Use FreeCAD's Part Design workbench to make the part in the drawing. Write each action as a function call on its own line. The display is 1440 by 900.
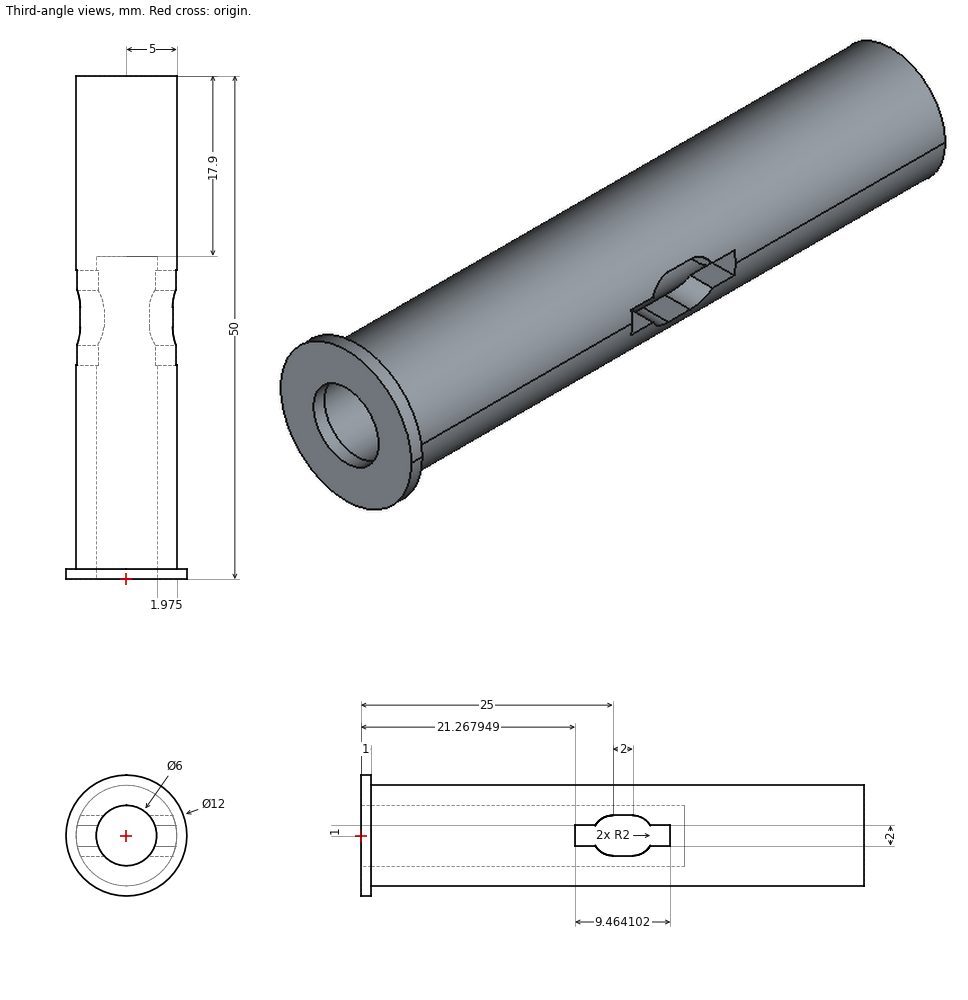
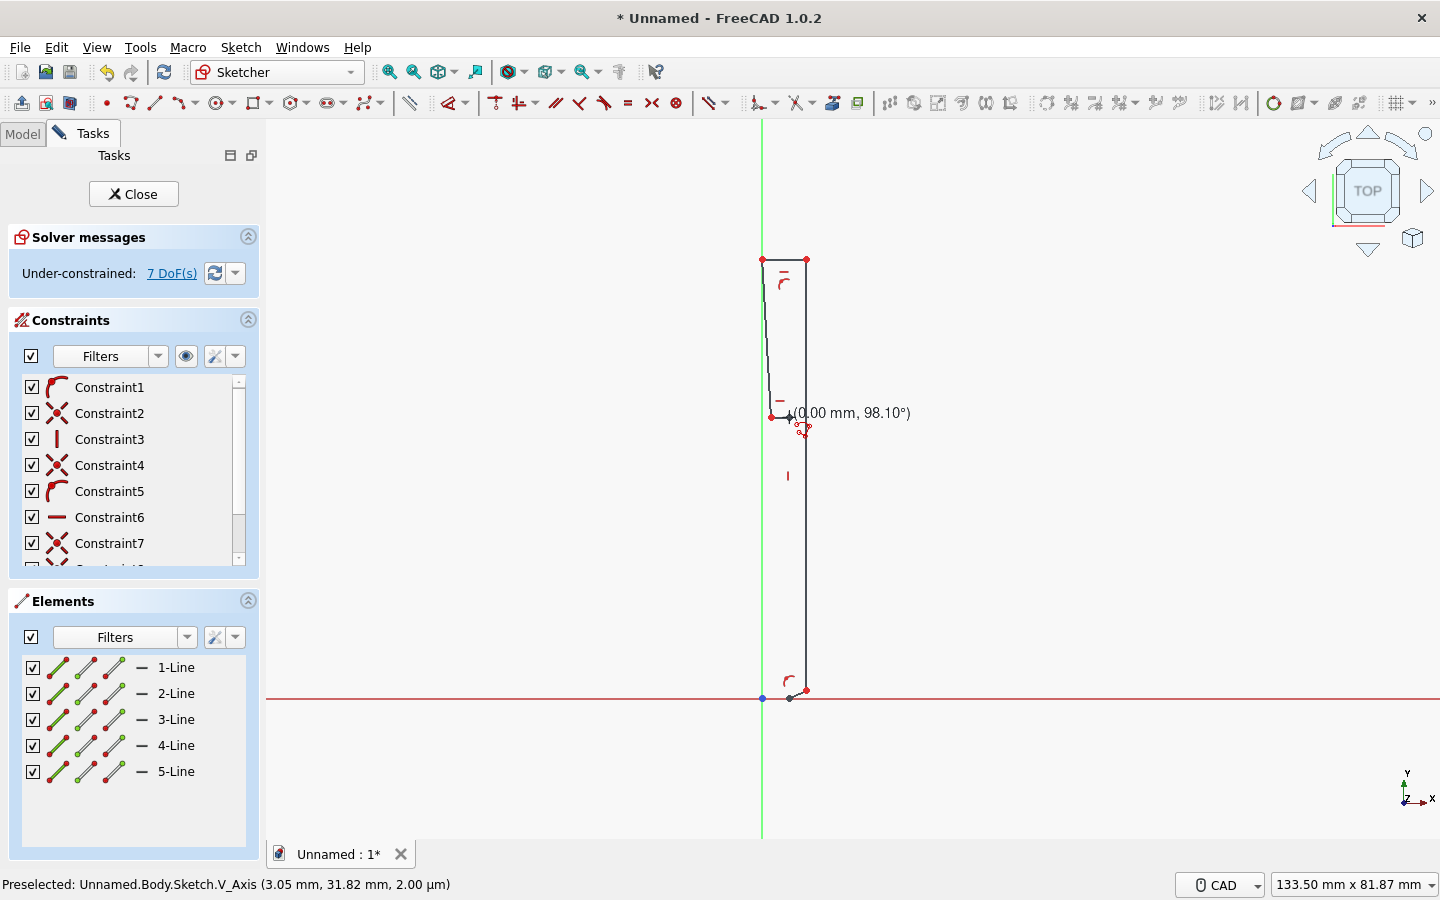
scroll(789, 699, up, 4)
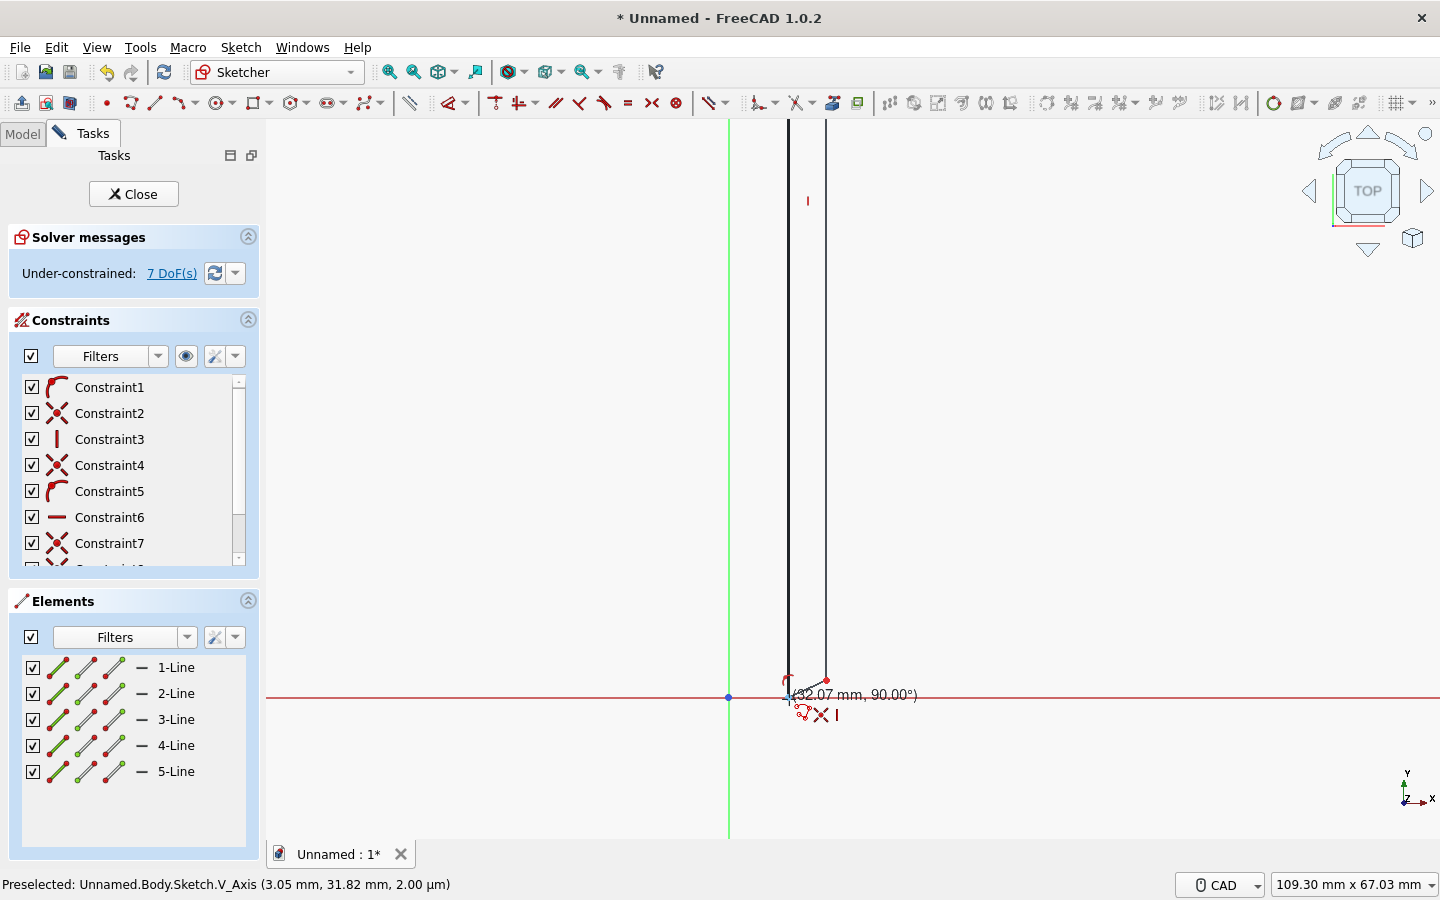
click(788, 698)
key(Escape)
key(Escape)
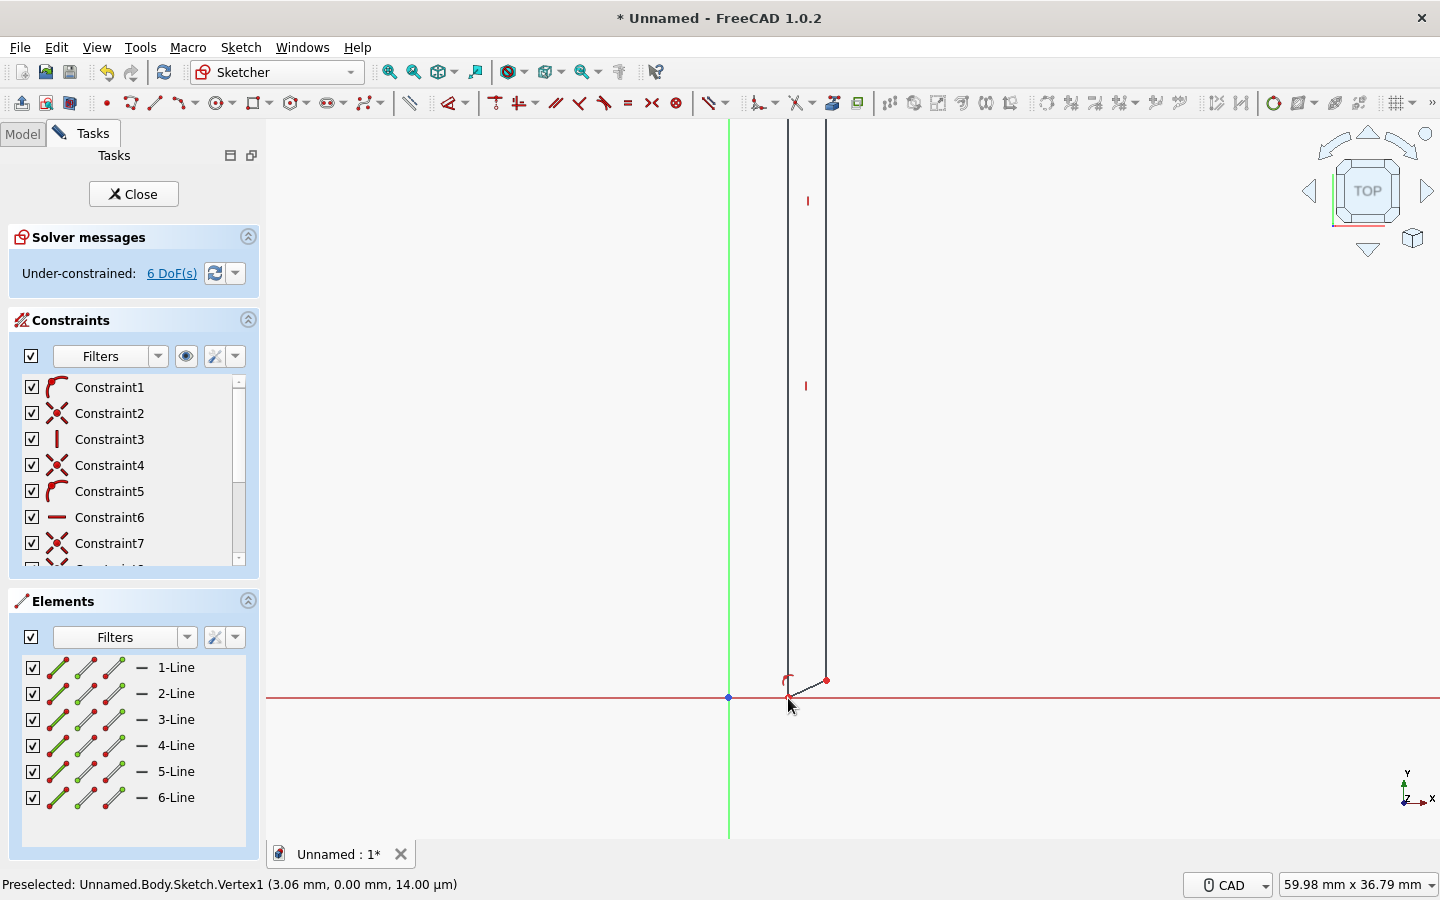
click(815, 685)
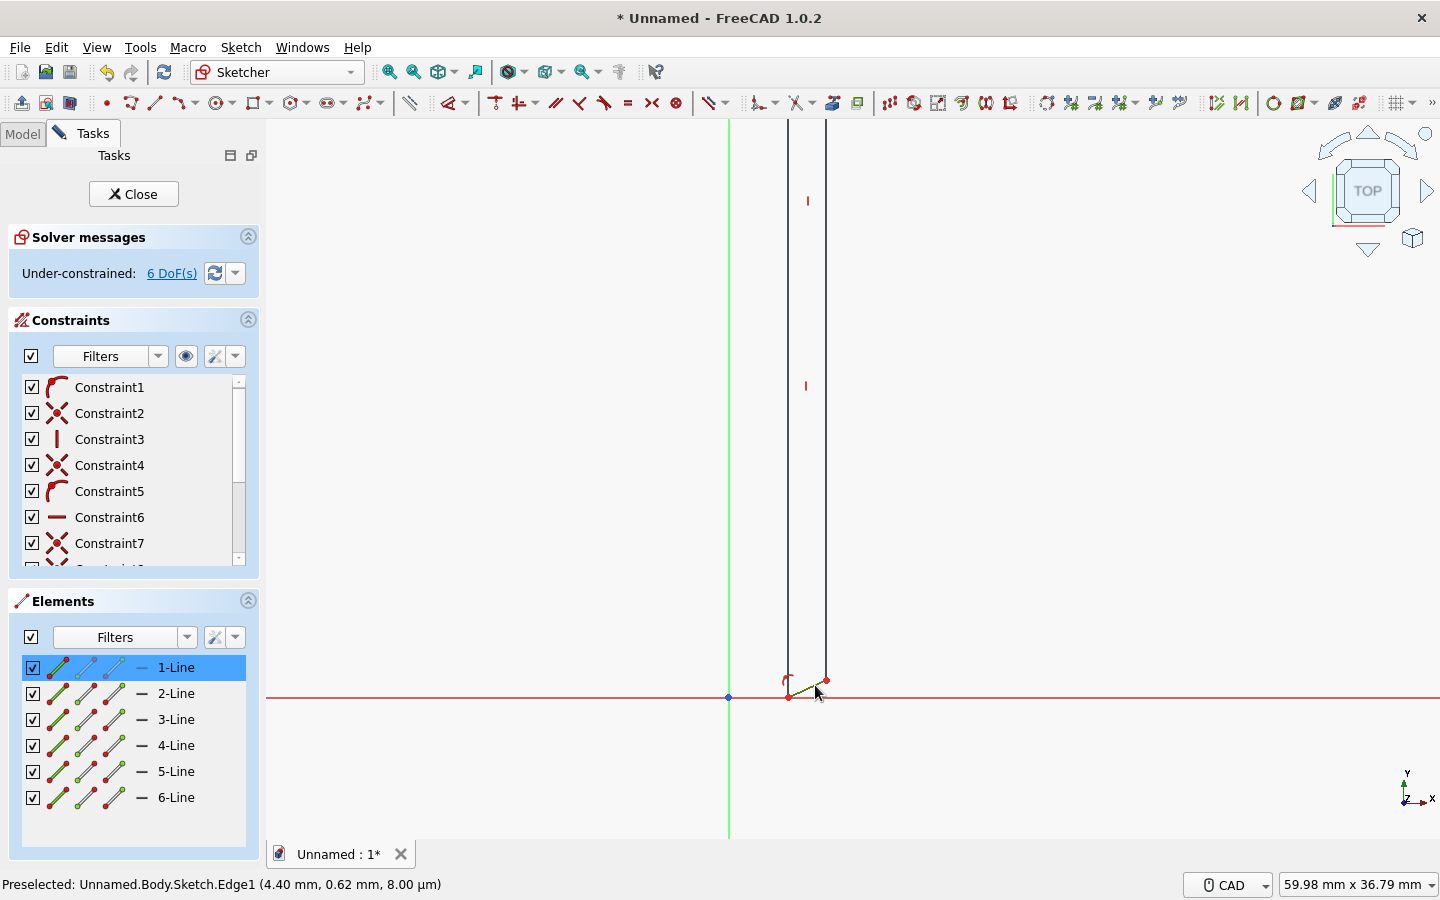
key(h)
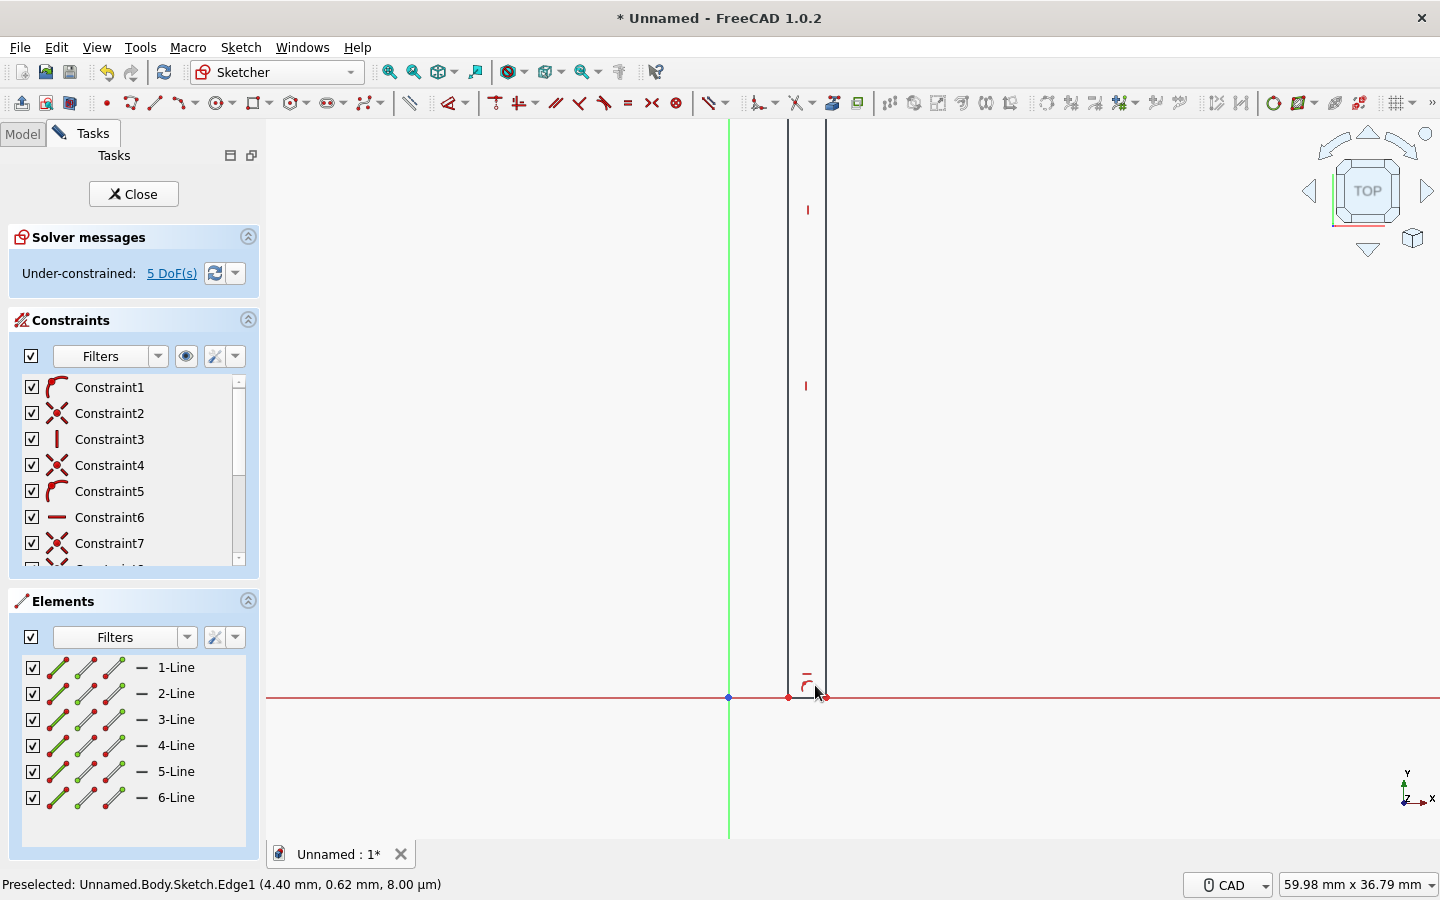
scroll(790, 700, down, 4)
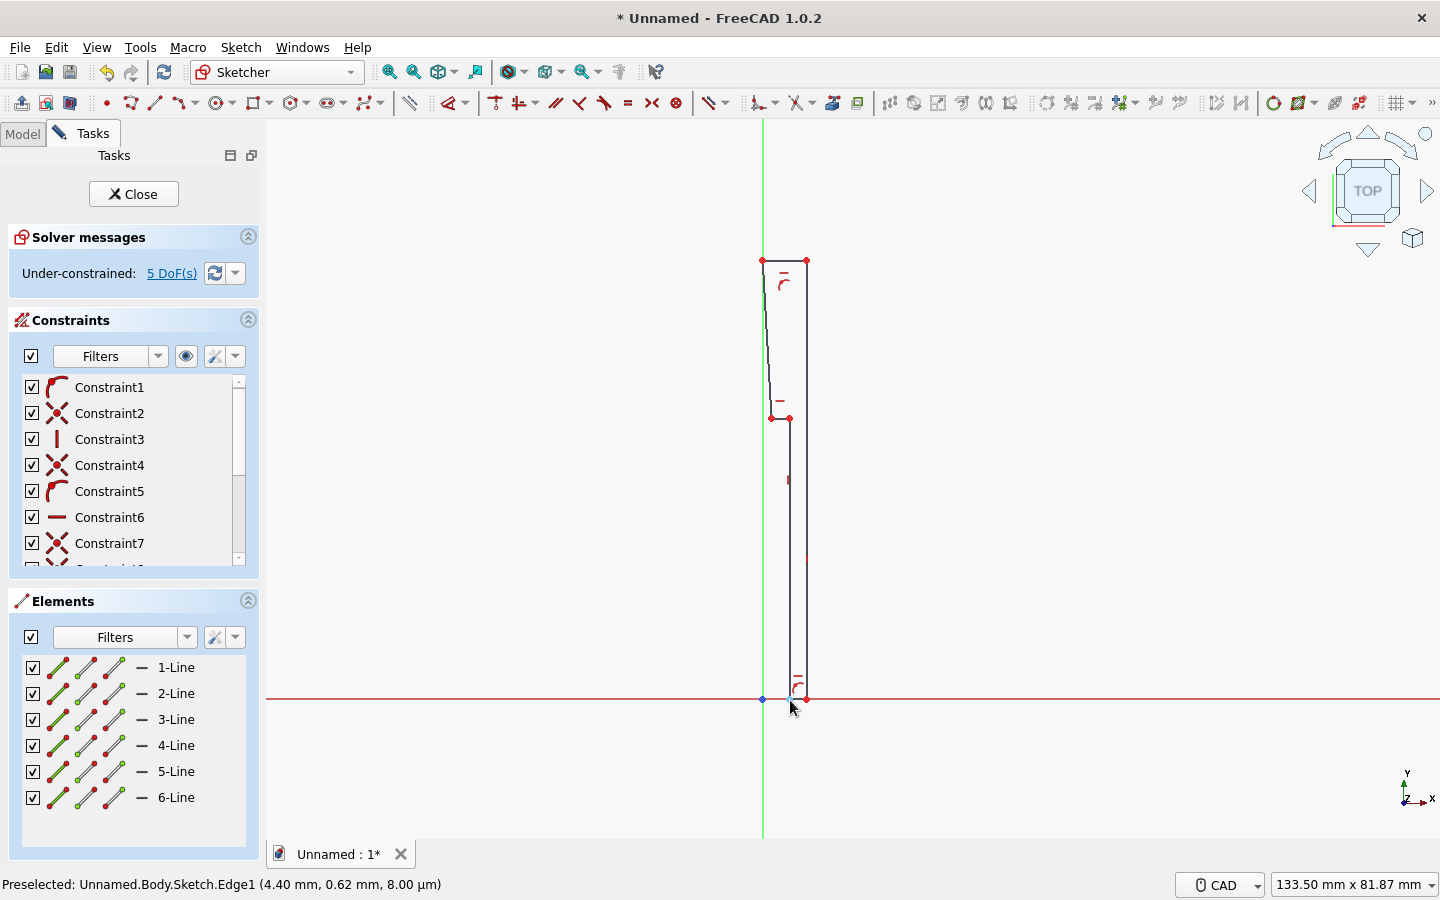
scroll(769, 371, up, 4)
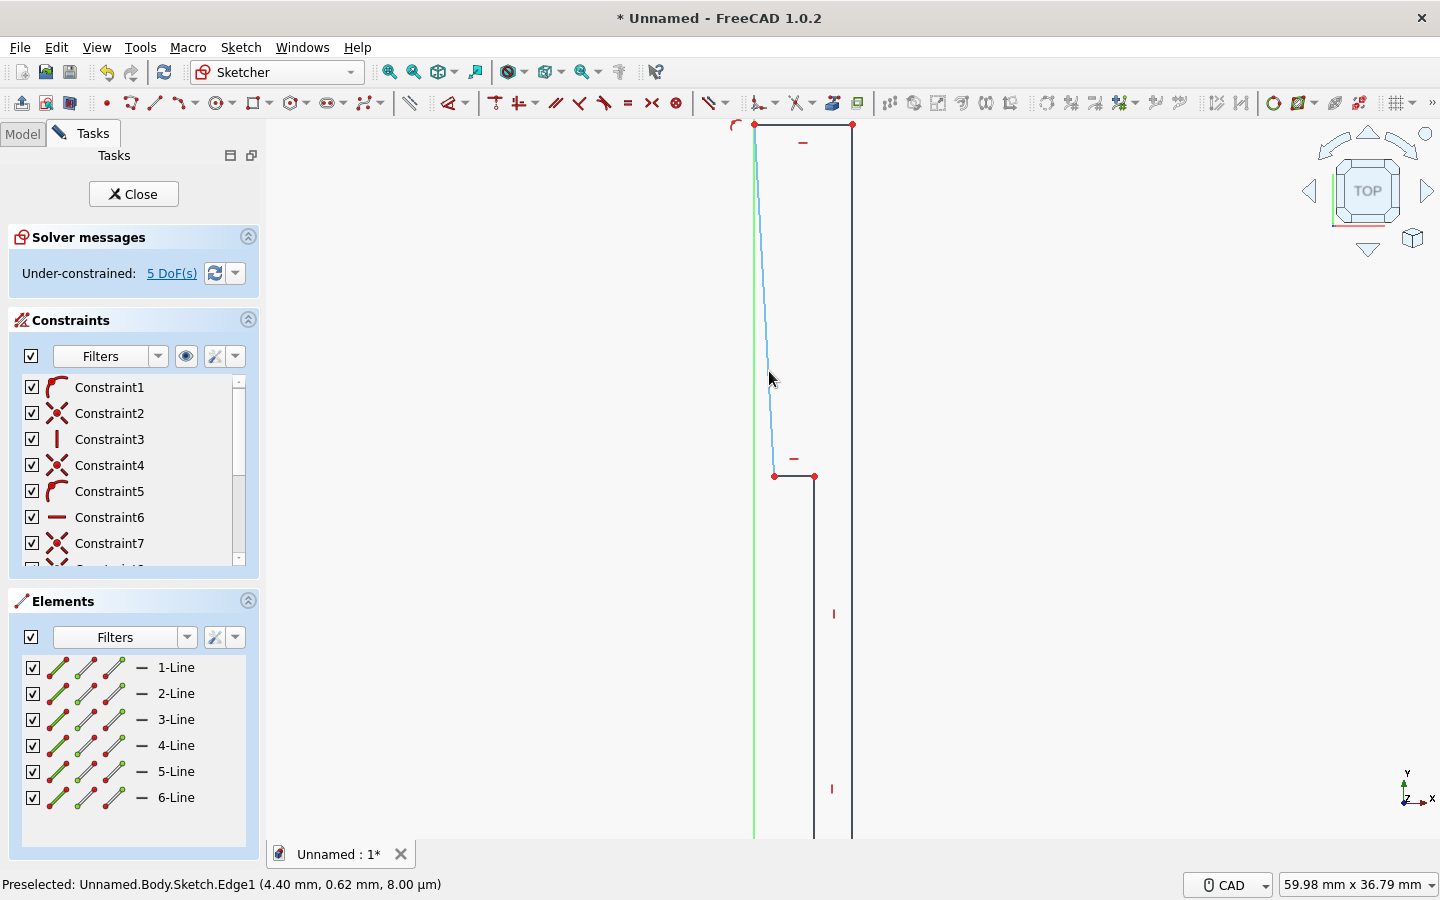
click(768, 371)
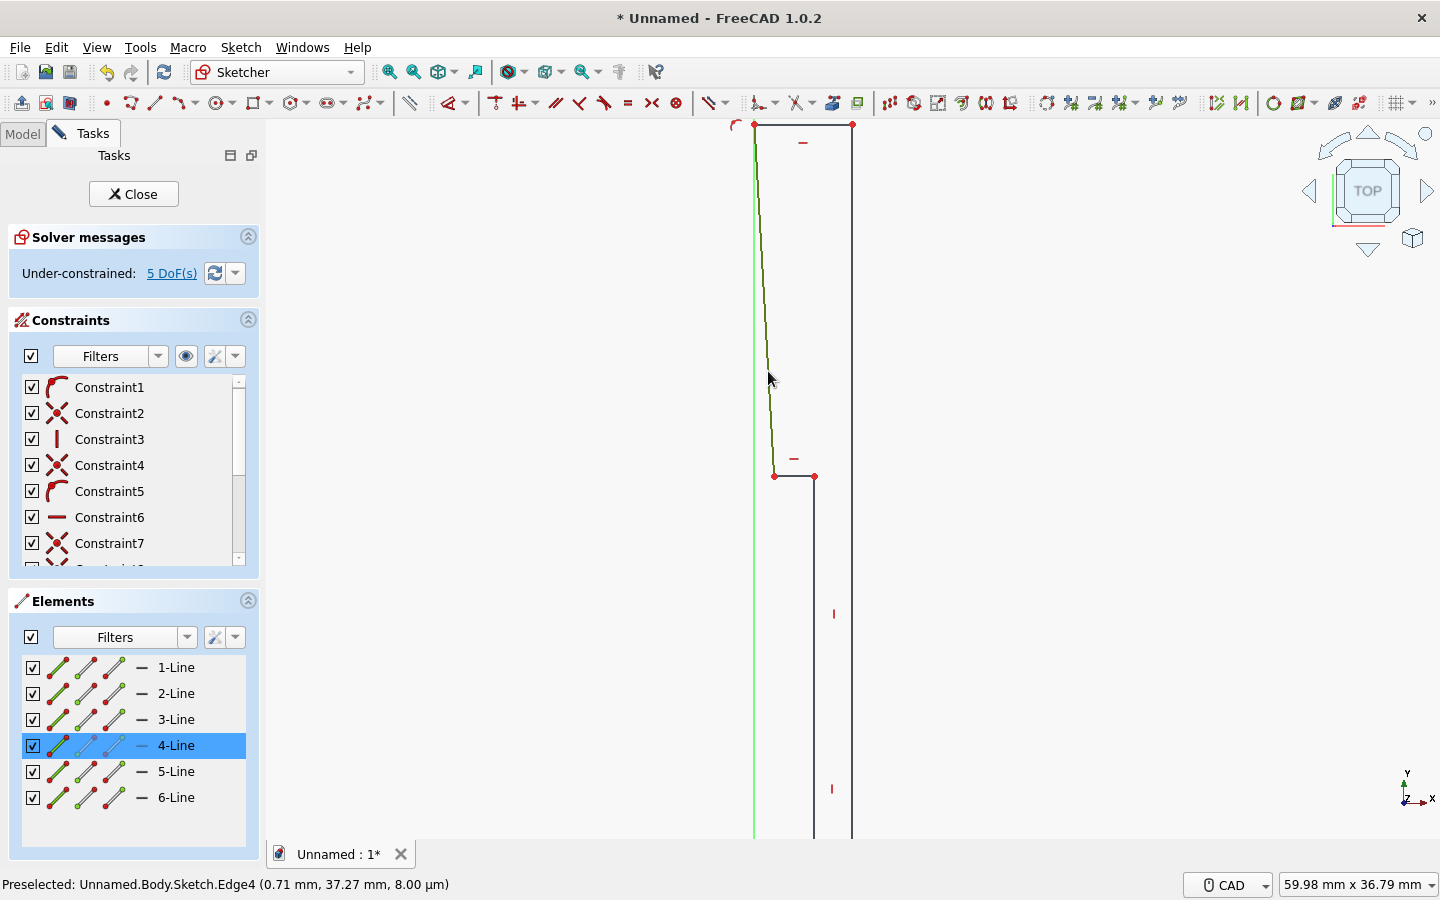
click(538, 104)